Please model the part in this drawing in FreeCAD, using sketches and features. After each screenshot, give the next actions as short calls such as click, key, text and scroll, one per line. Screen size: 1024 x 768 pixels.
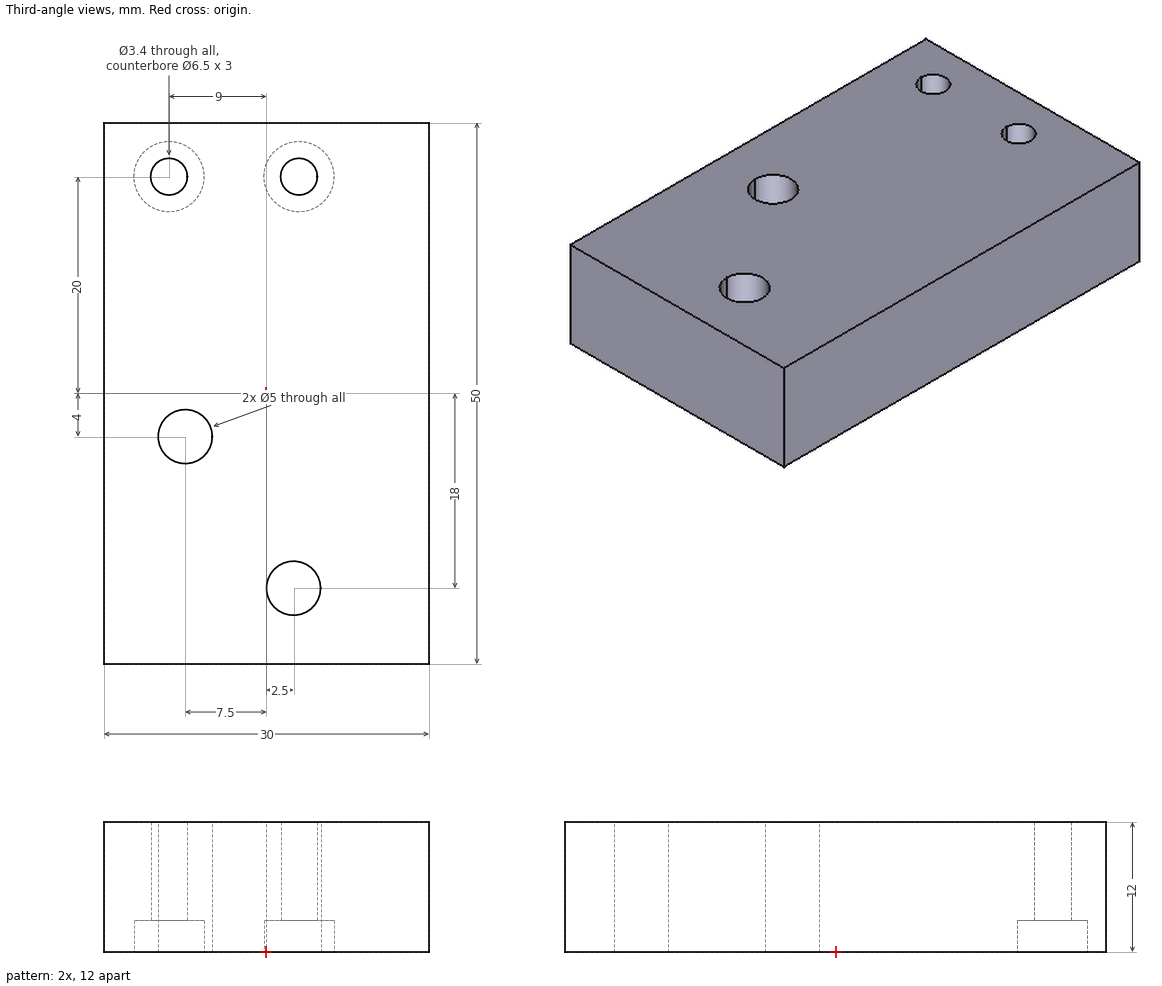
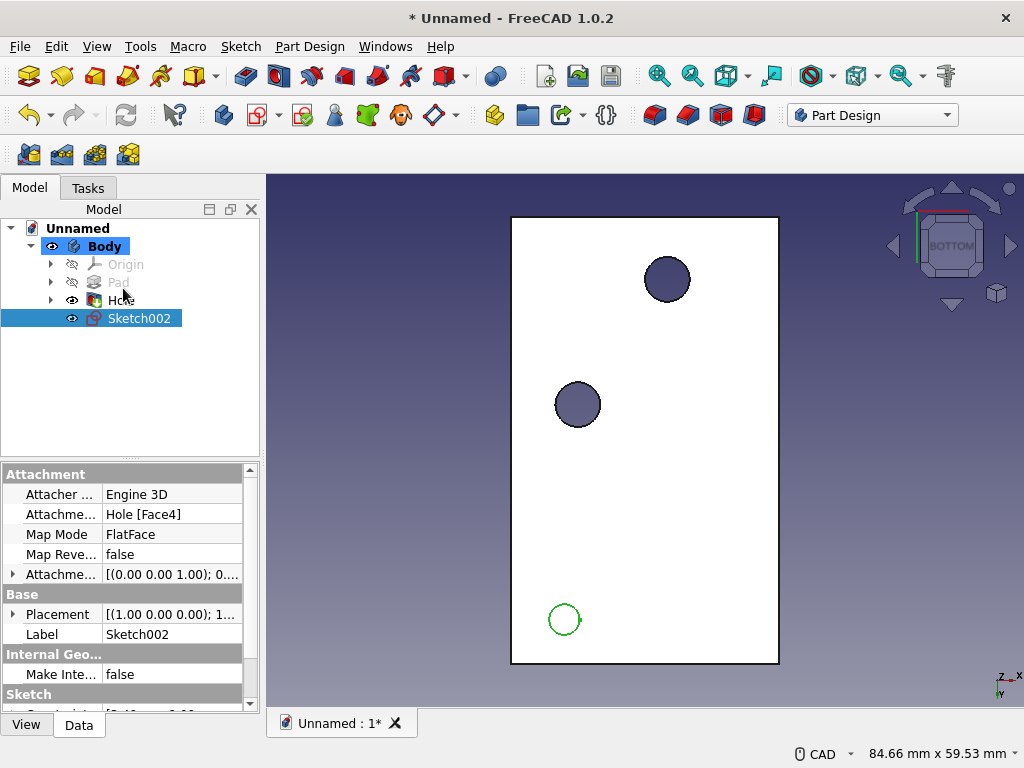
click(279, 76)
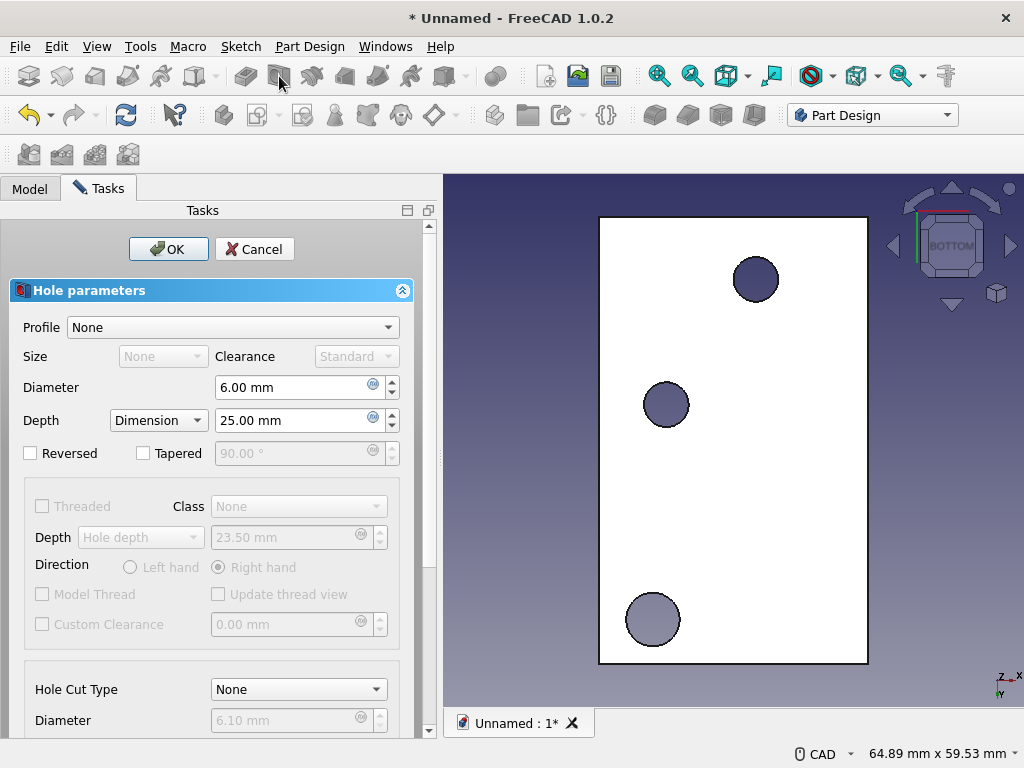
triple_click(300, 388)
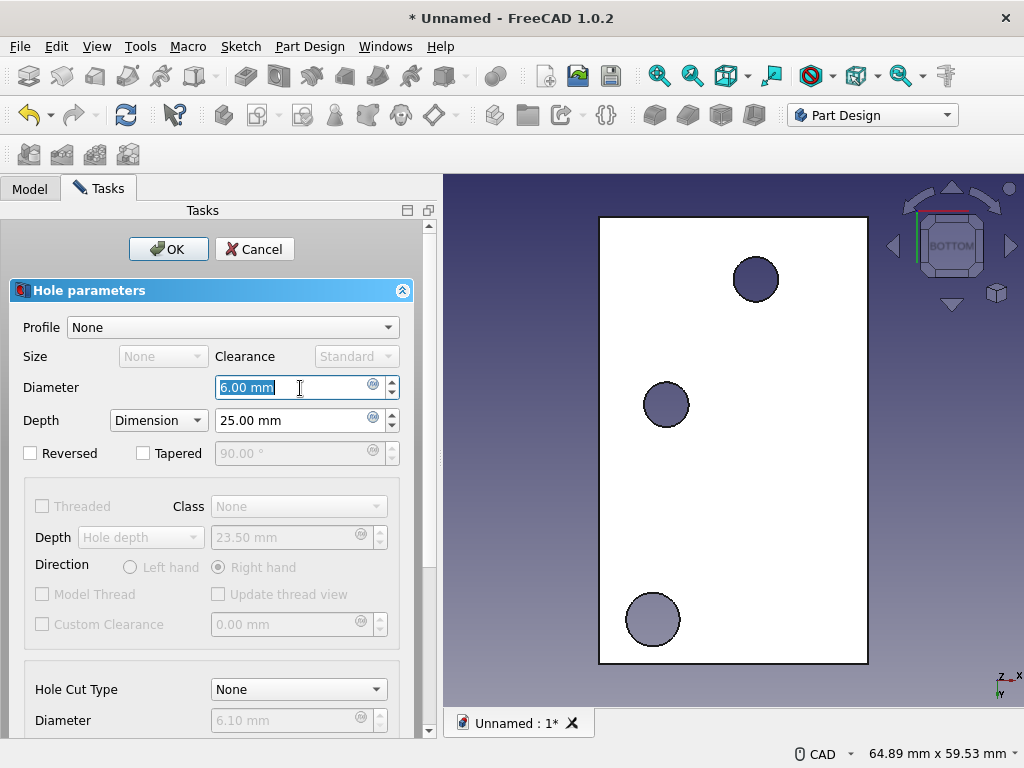
text(3.4)
key(Tab)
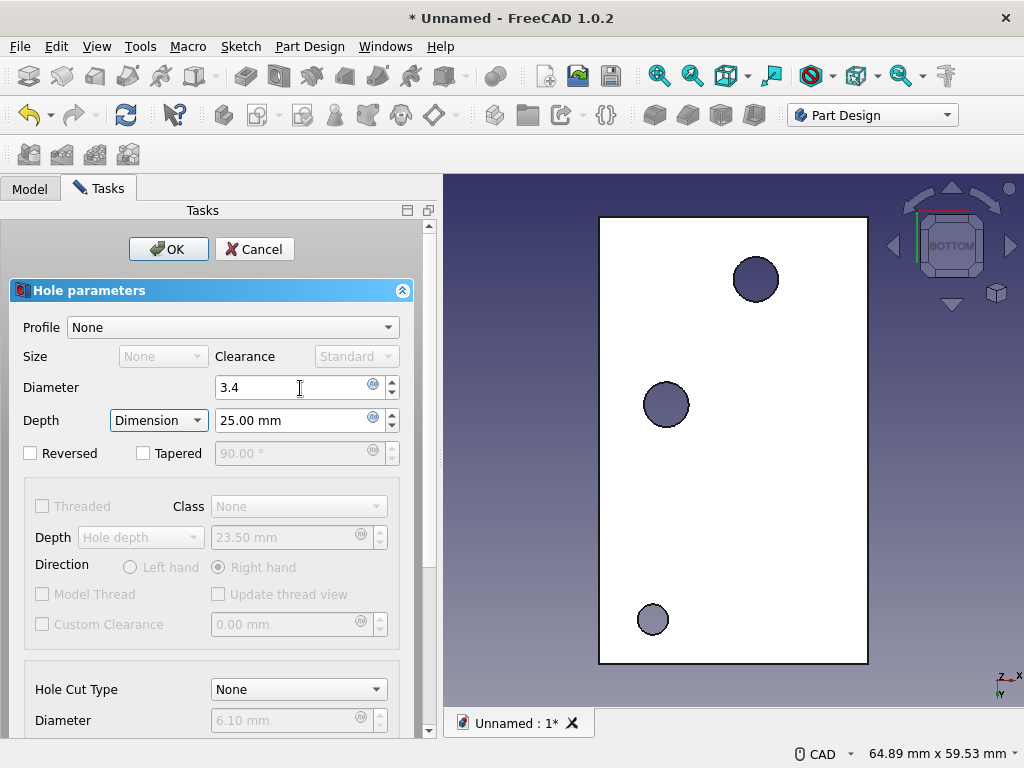
click(160, 420)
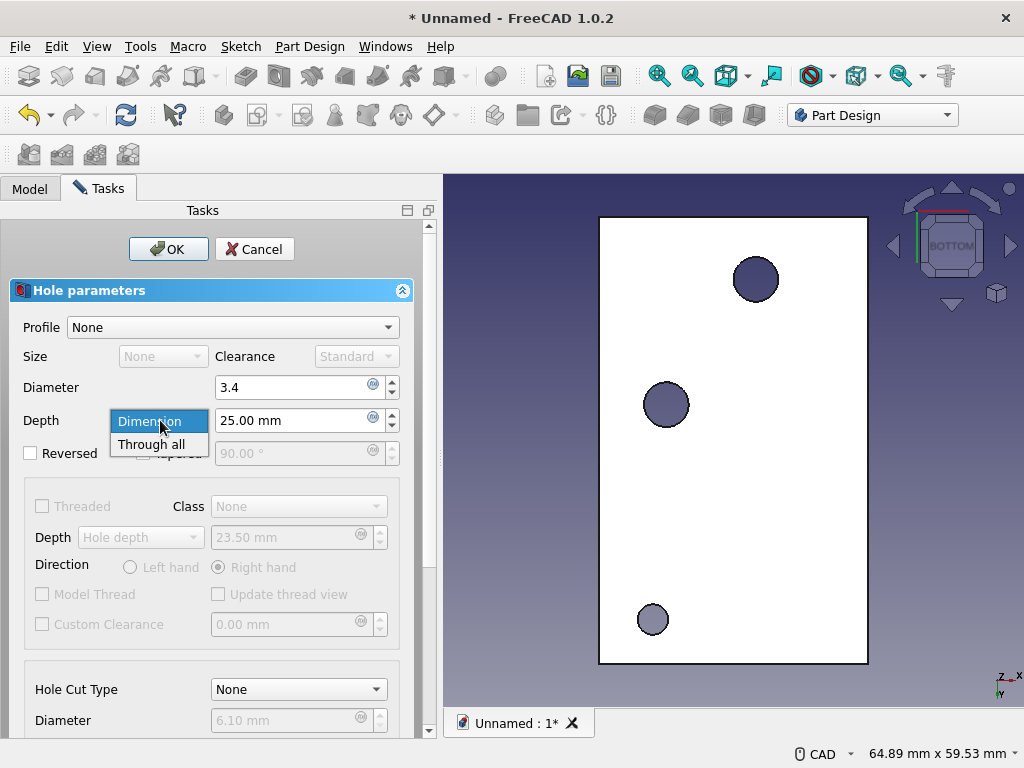
click(158, 444)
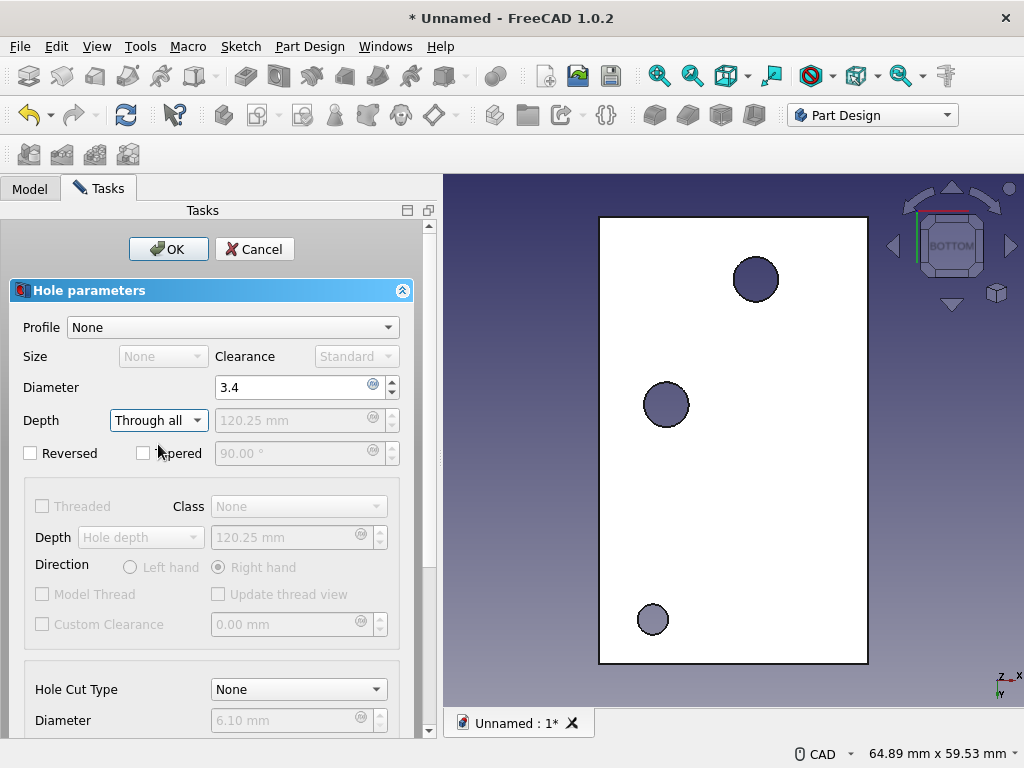
click(300, 690)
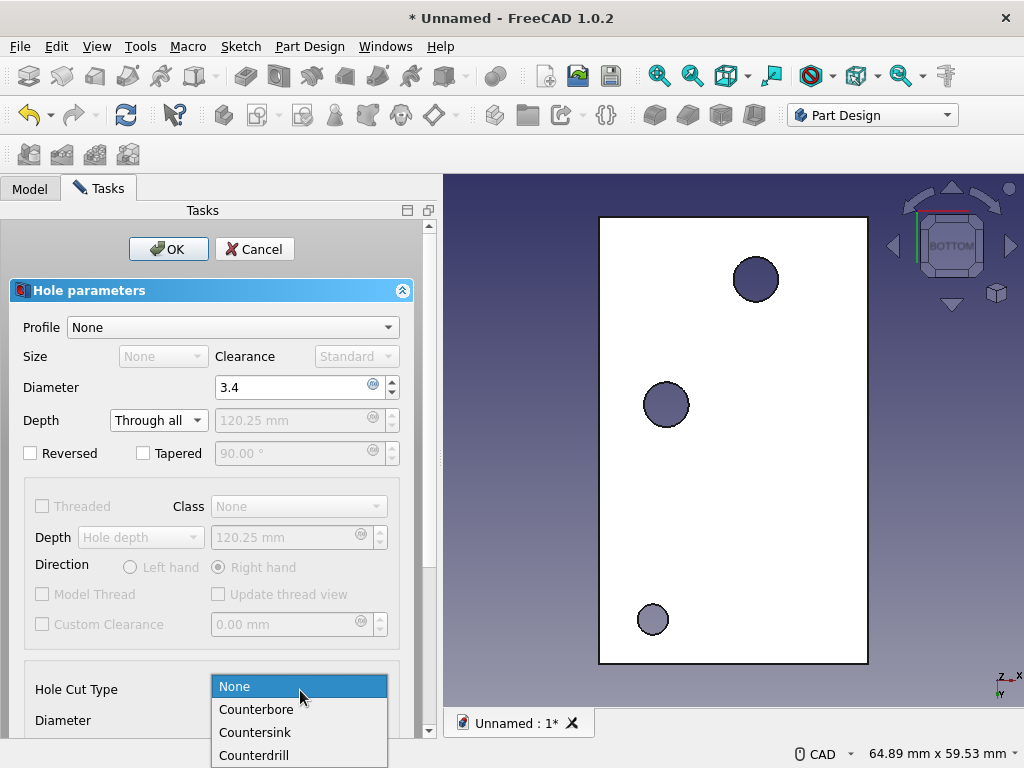
click(298, 710)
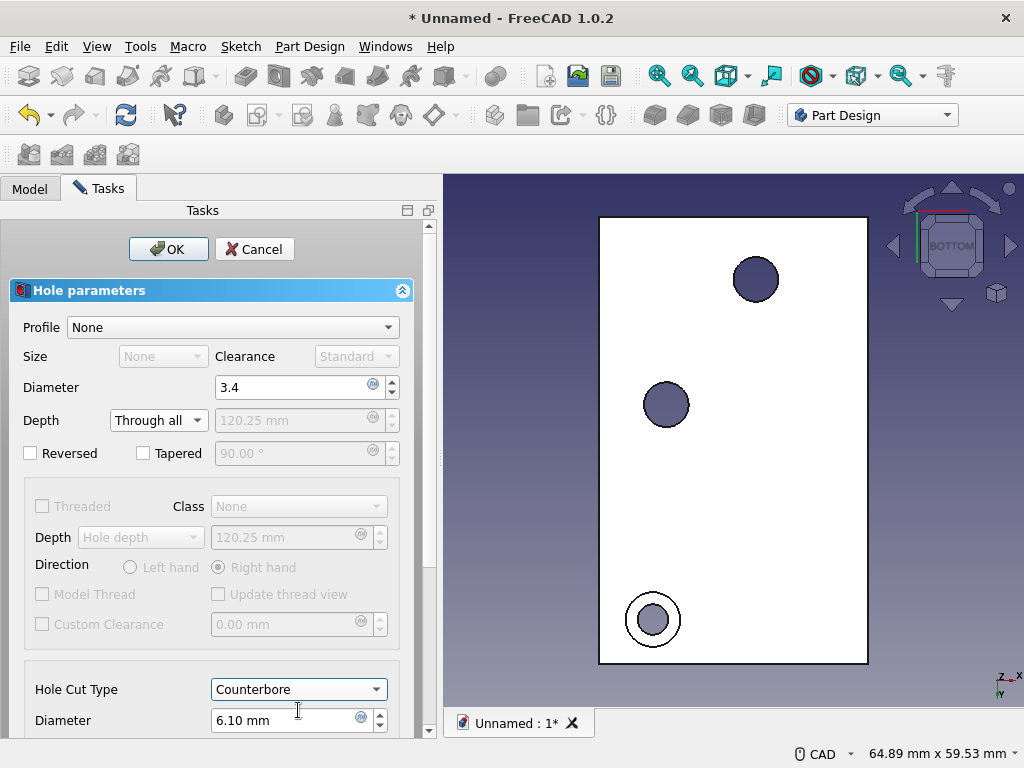
triple_click(292, 720)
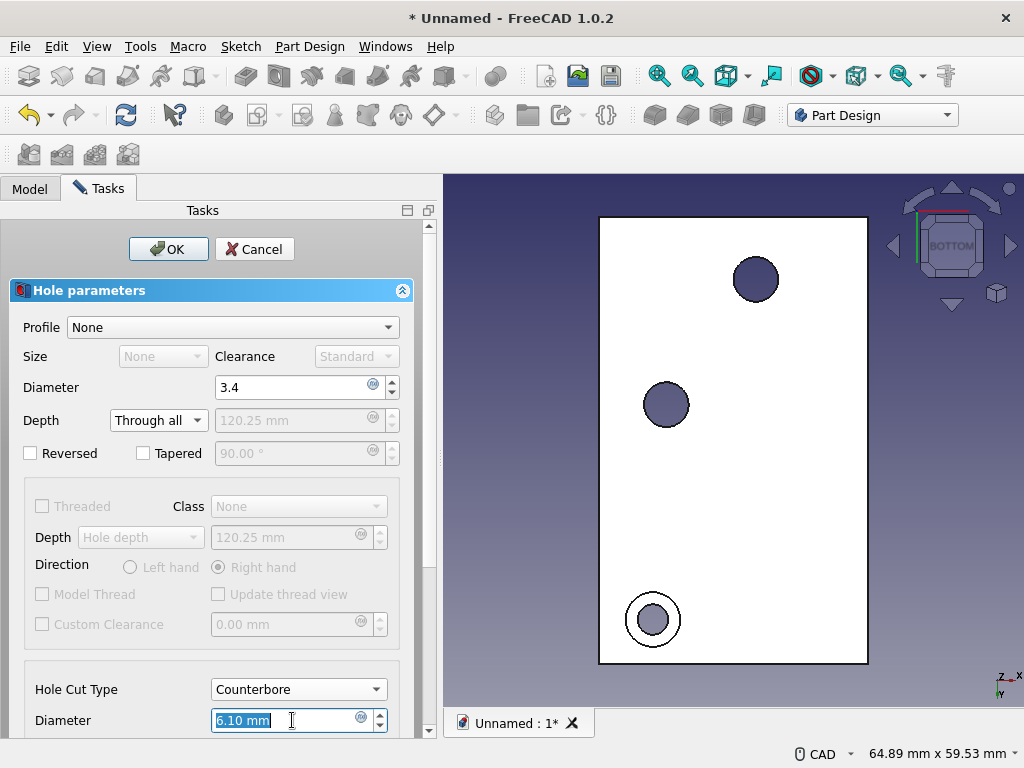
text(6.5)
key(Tab)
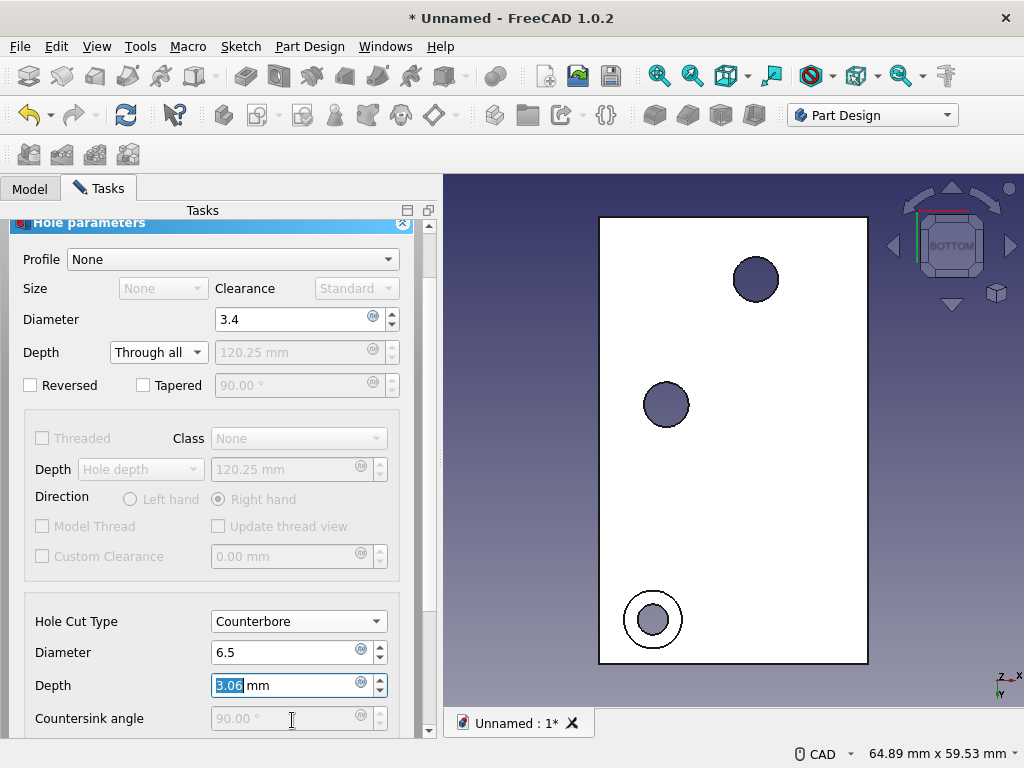
text(3)
key(Tab)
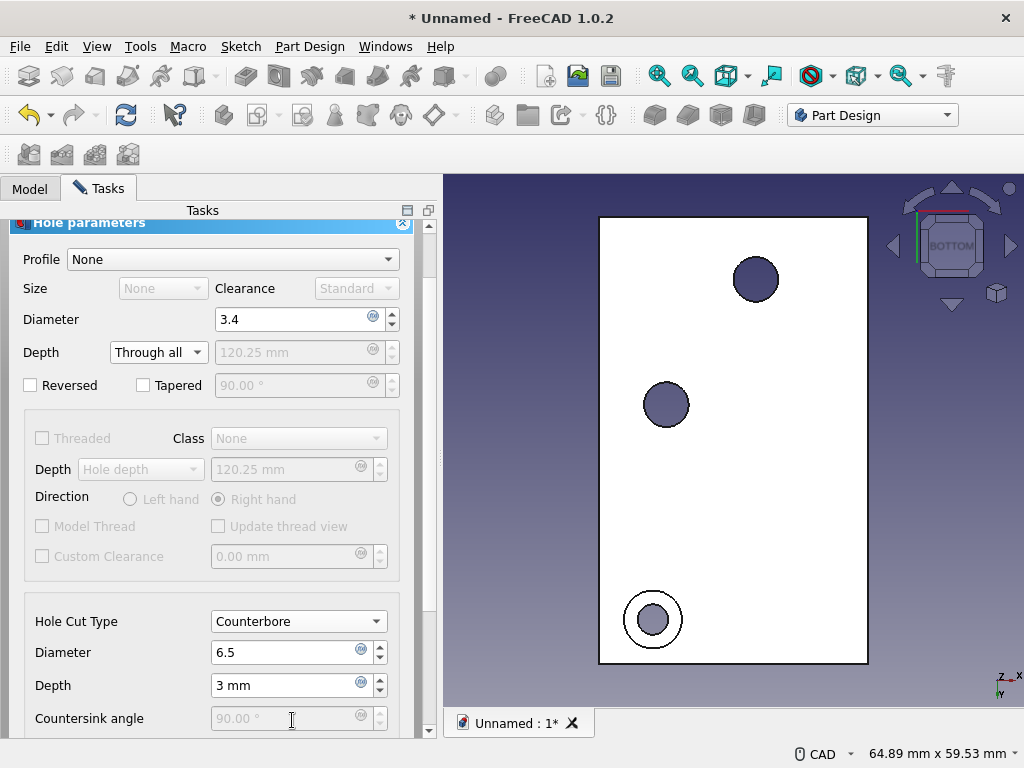
scroll(429, 479, up, 2)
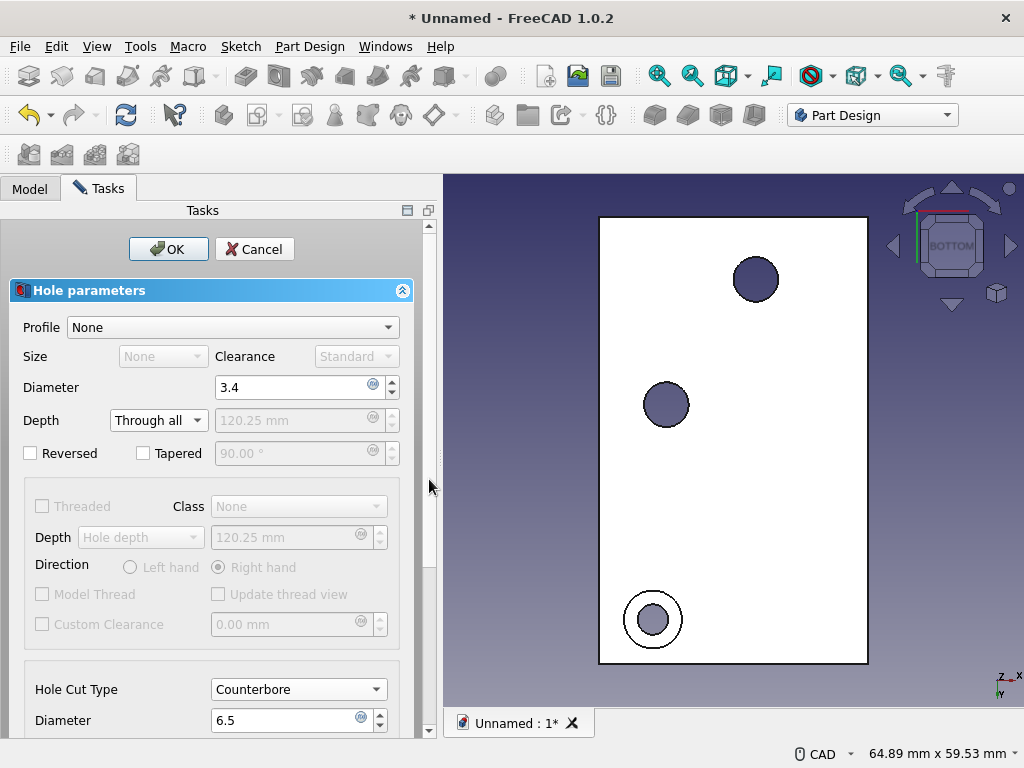
click(169, 249)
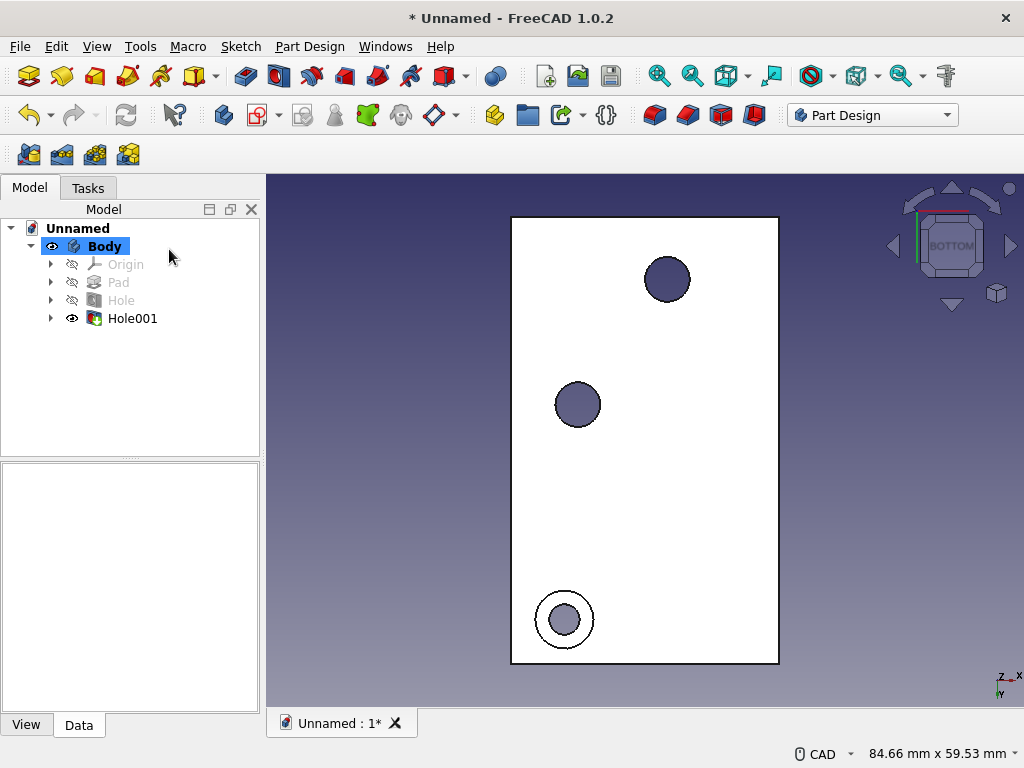
click(117, 318)